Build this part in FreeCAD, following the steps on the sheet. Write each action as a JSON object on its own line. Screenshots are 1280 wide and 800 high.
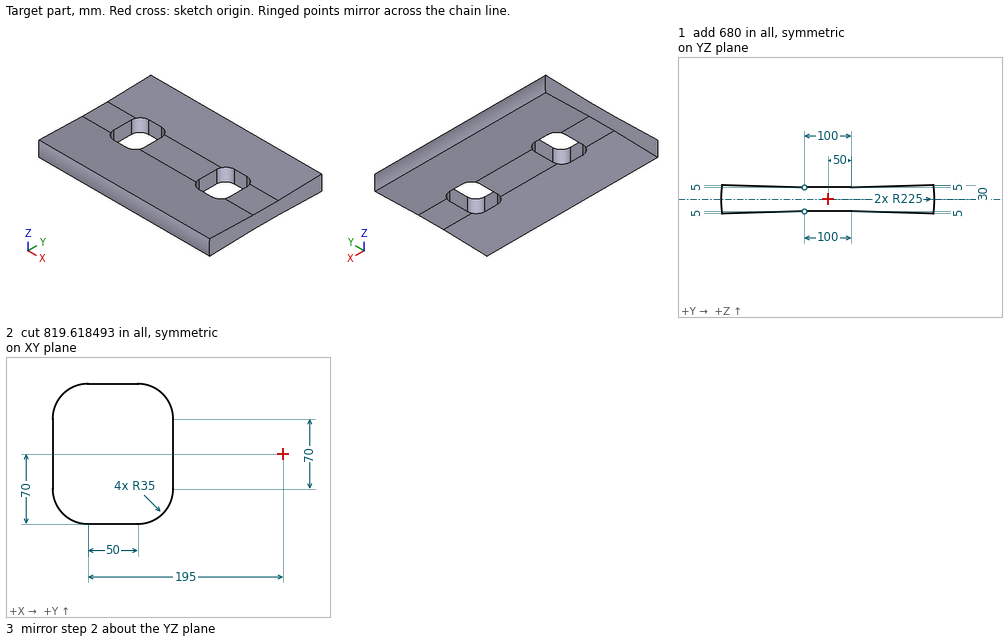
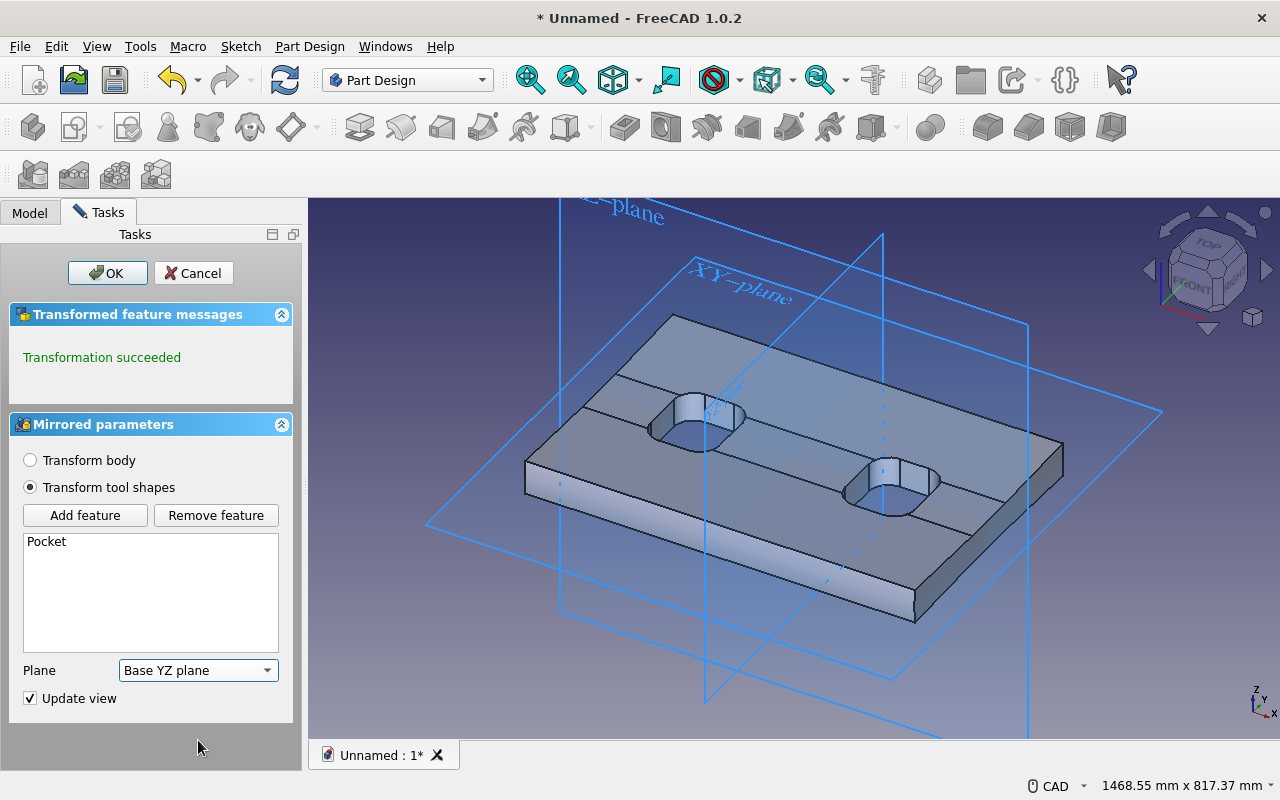
{"action": "left_click", "coordinate": [108, 273]}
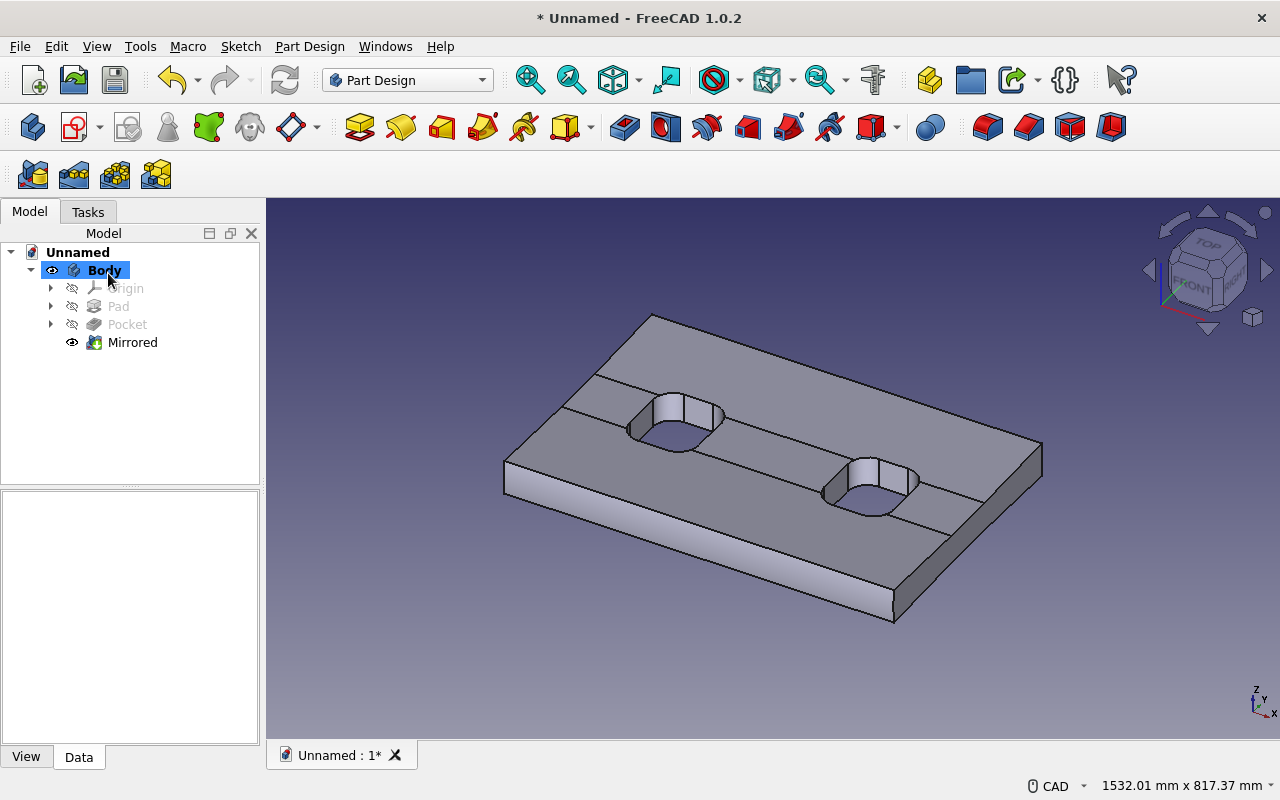
{"action": "key", "text": "0"}